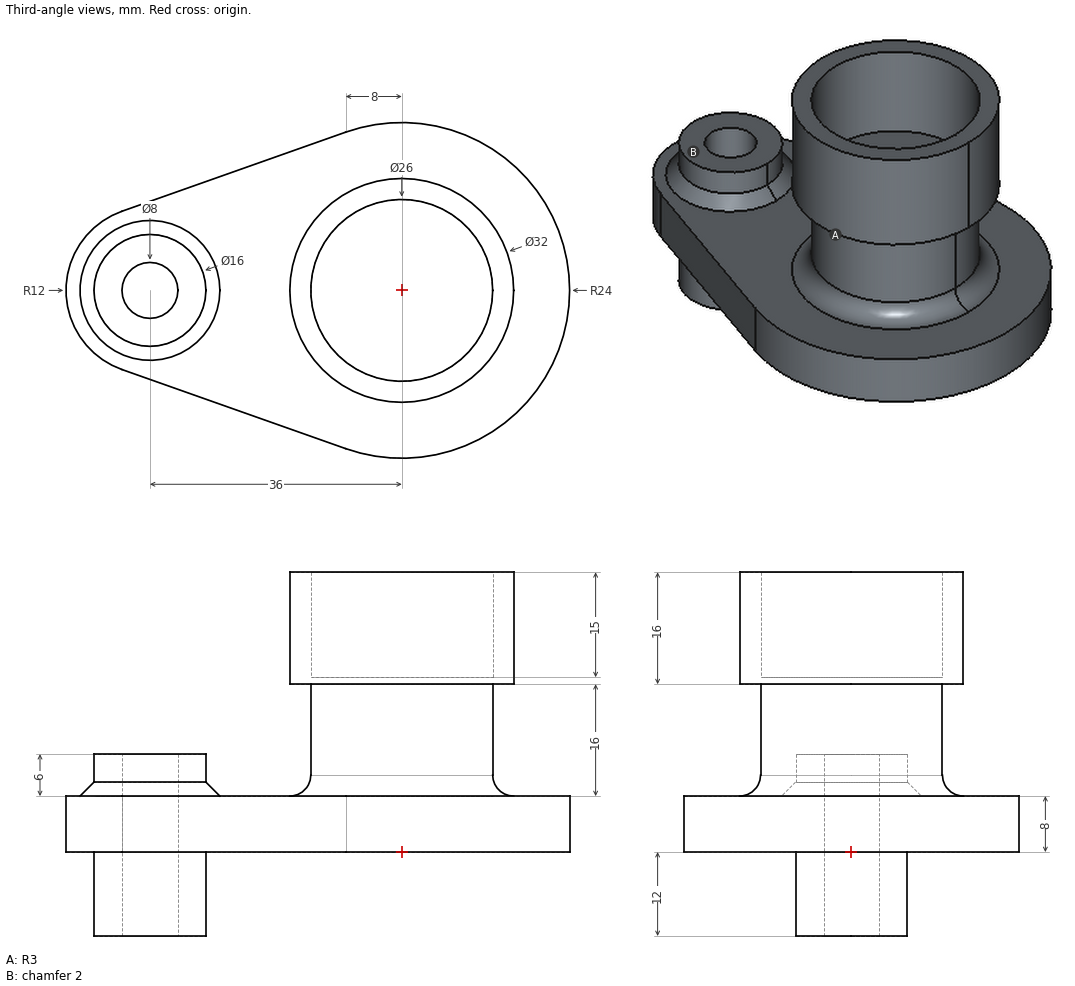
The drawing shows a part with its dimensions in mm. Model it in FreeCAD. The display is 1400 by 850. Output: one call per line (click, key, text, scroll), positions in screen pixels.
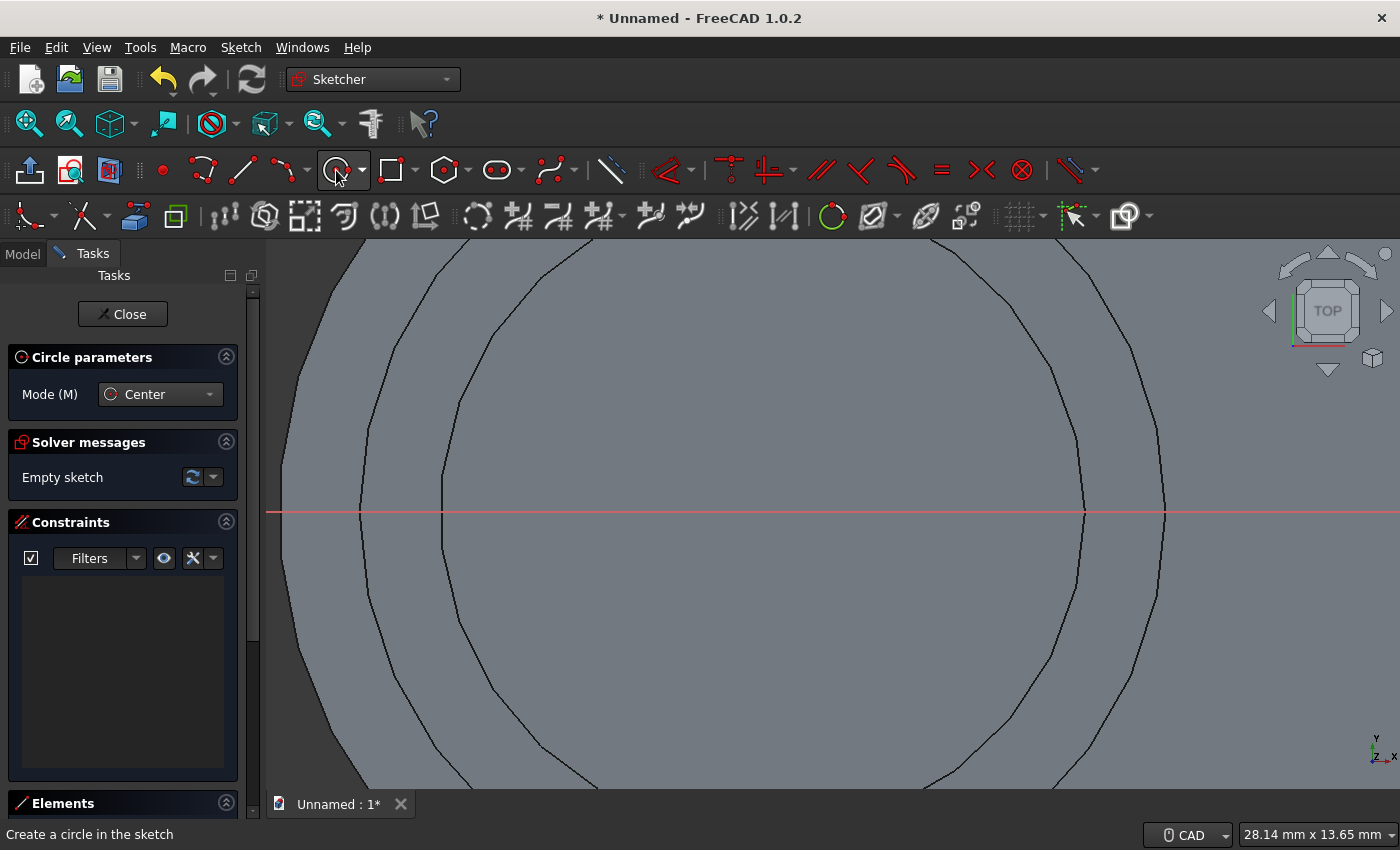
click(763, 512)
move(877, 398)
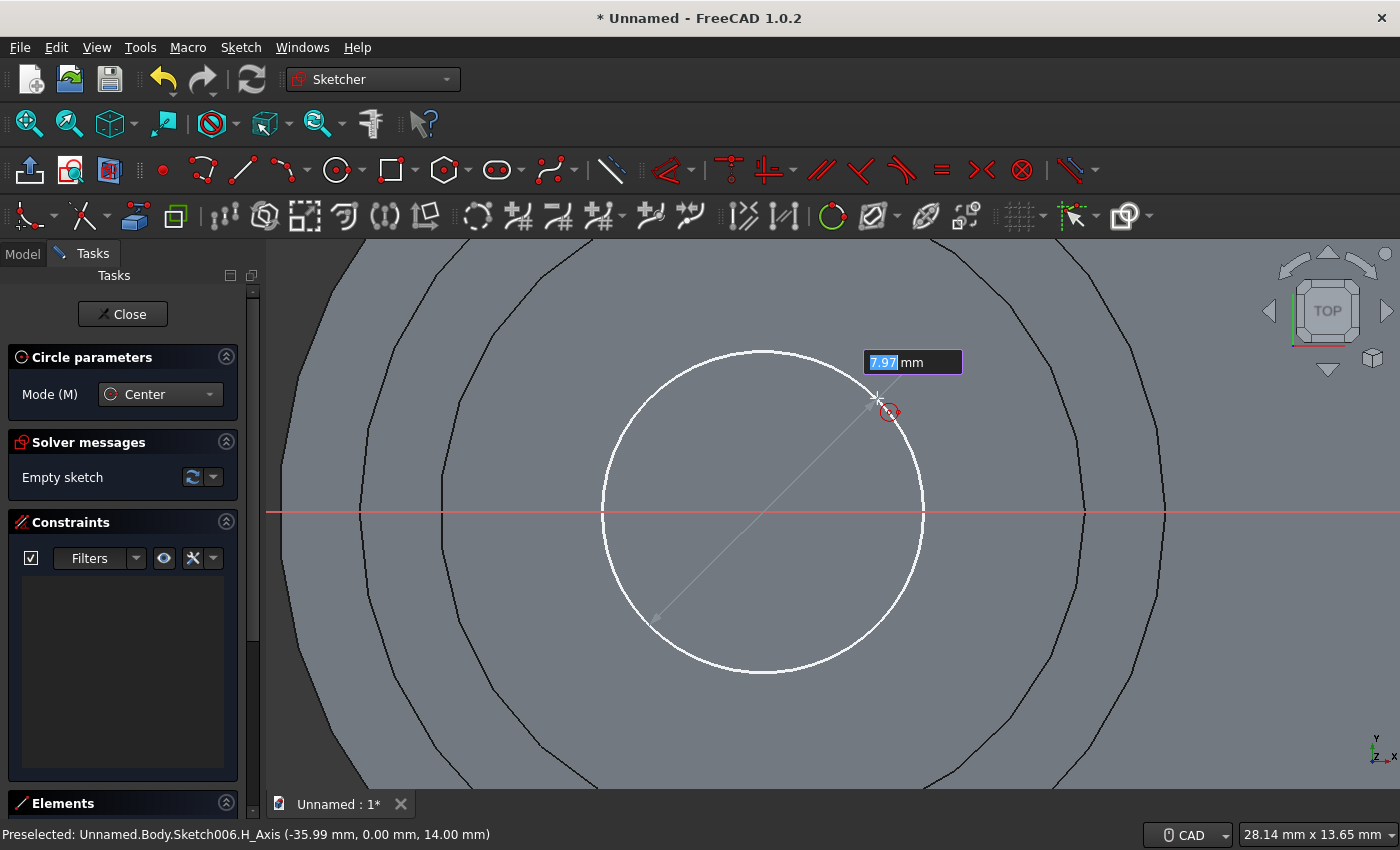
text(8)
key(Return)
key(Escape)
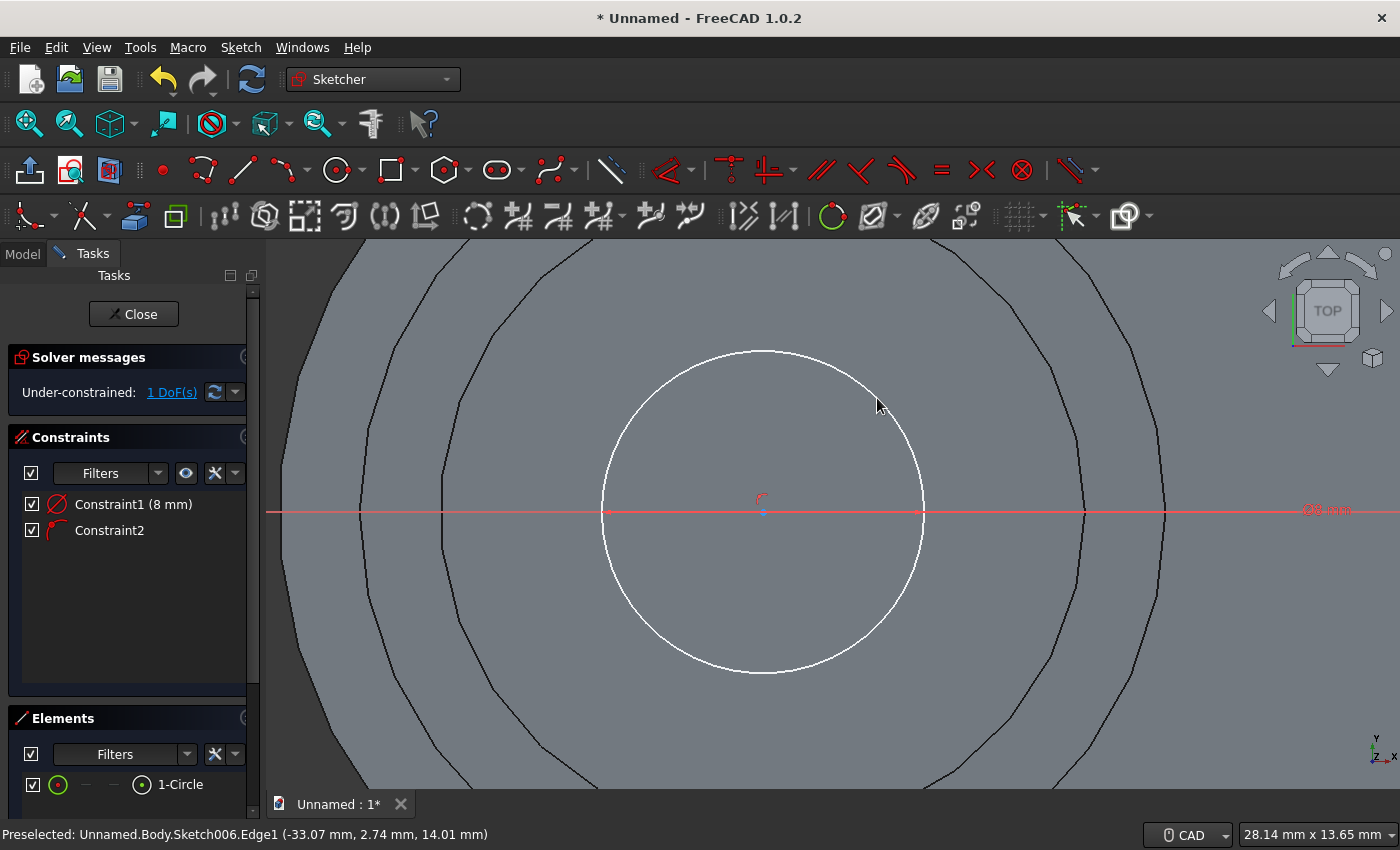
click(666, 170)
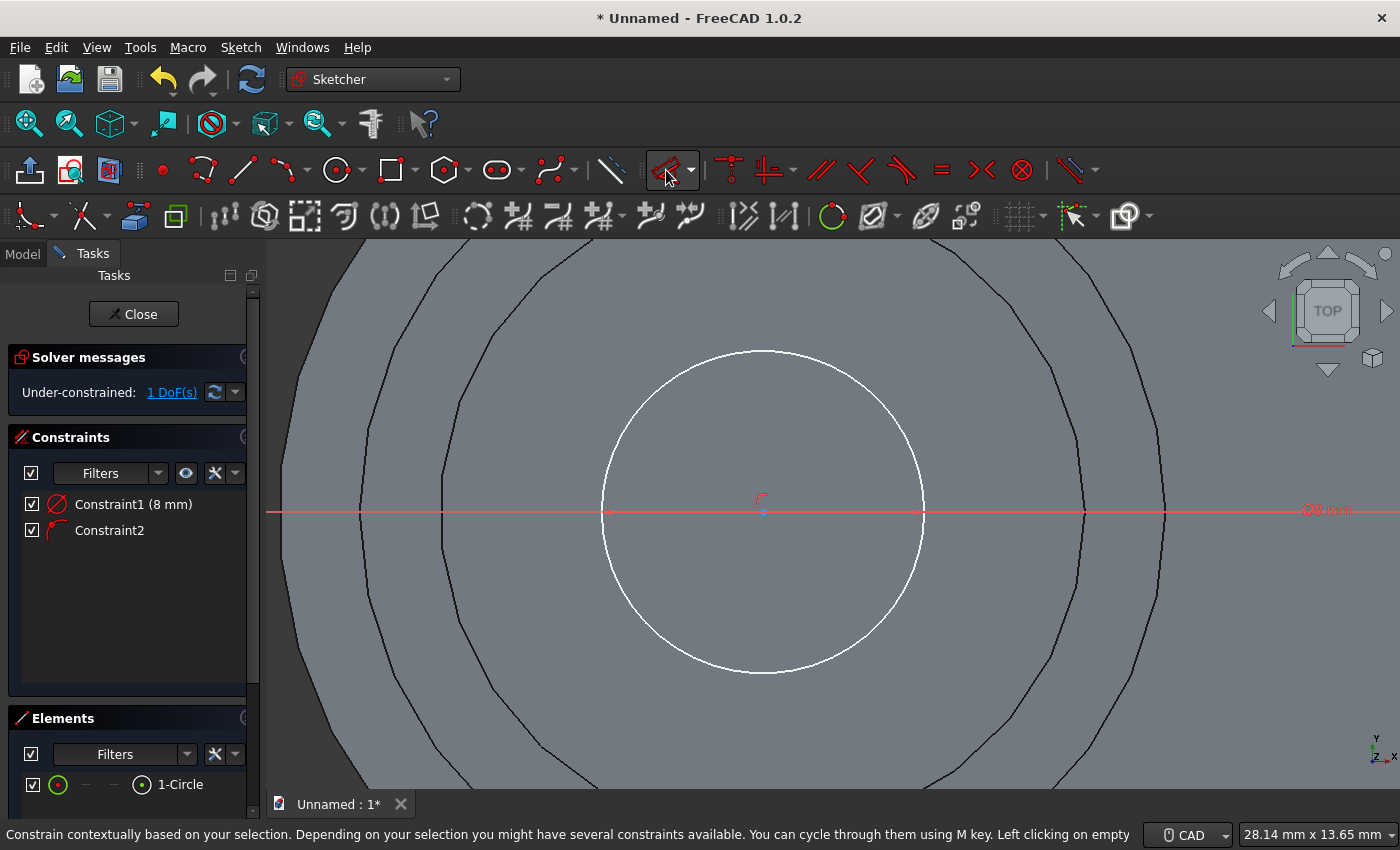
click(763, 512)
click(999, 546)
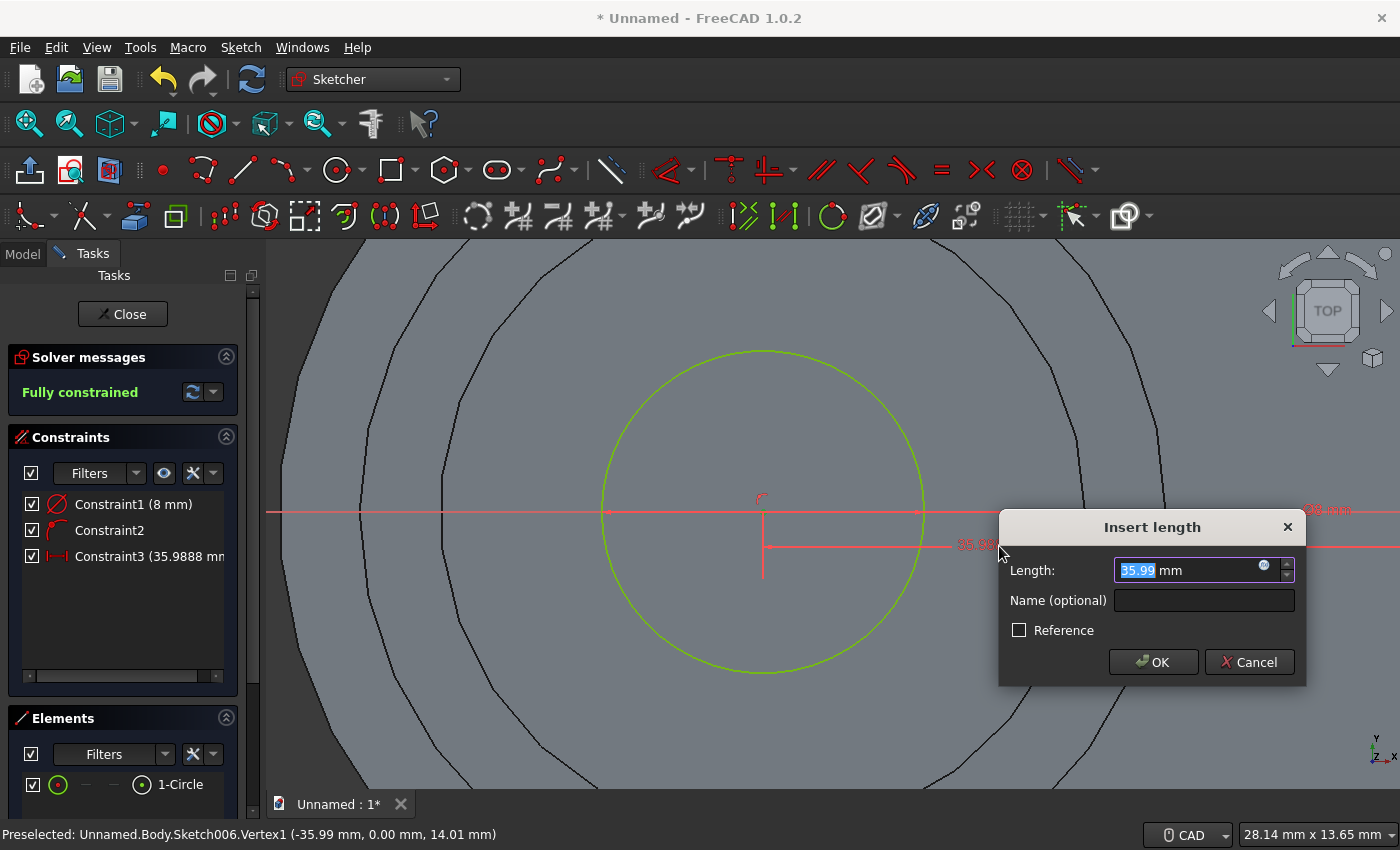
text(36)
key(Return)
key(Escape)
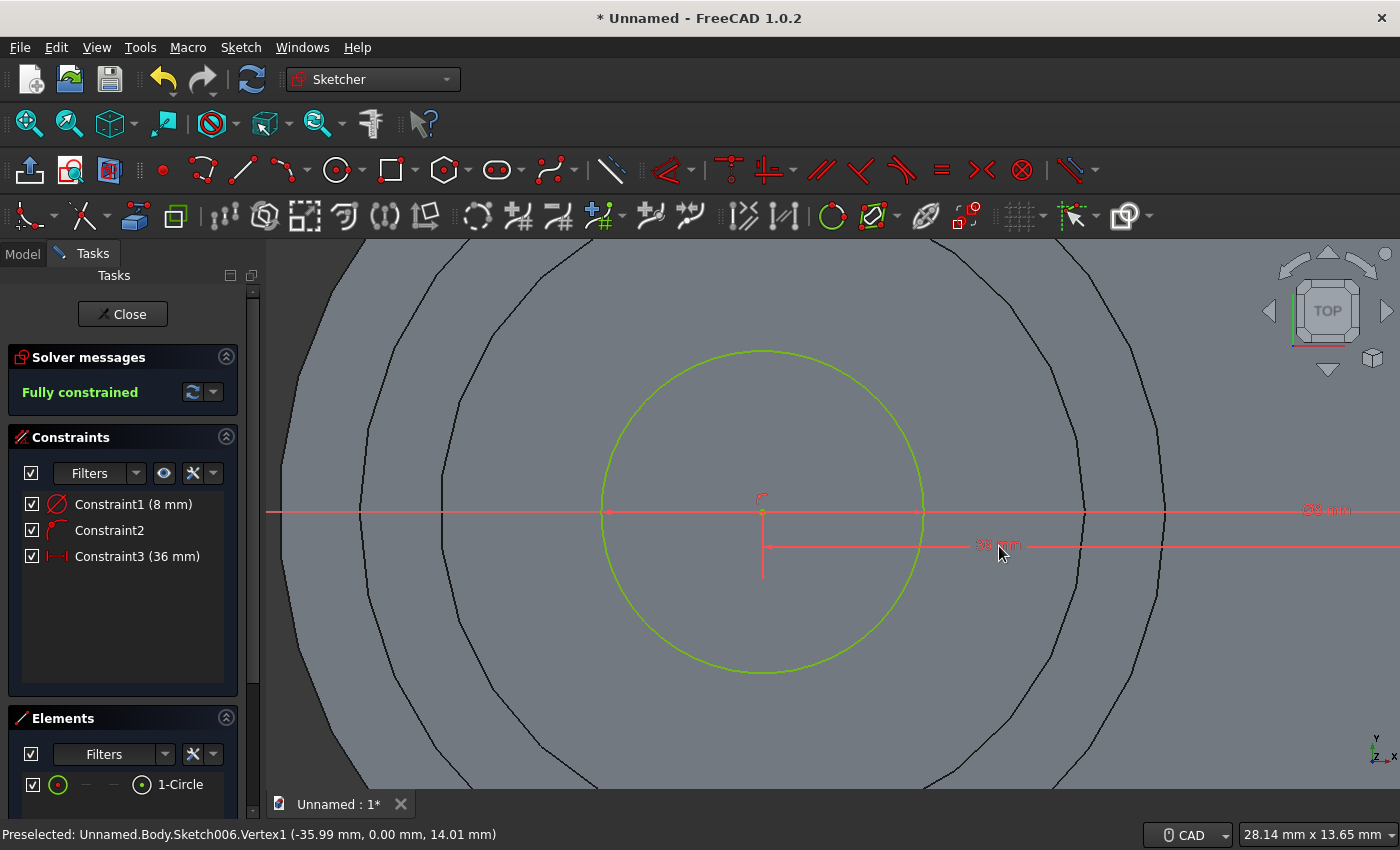
click(123, 314)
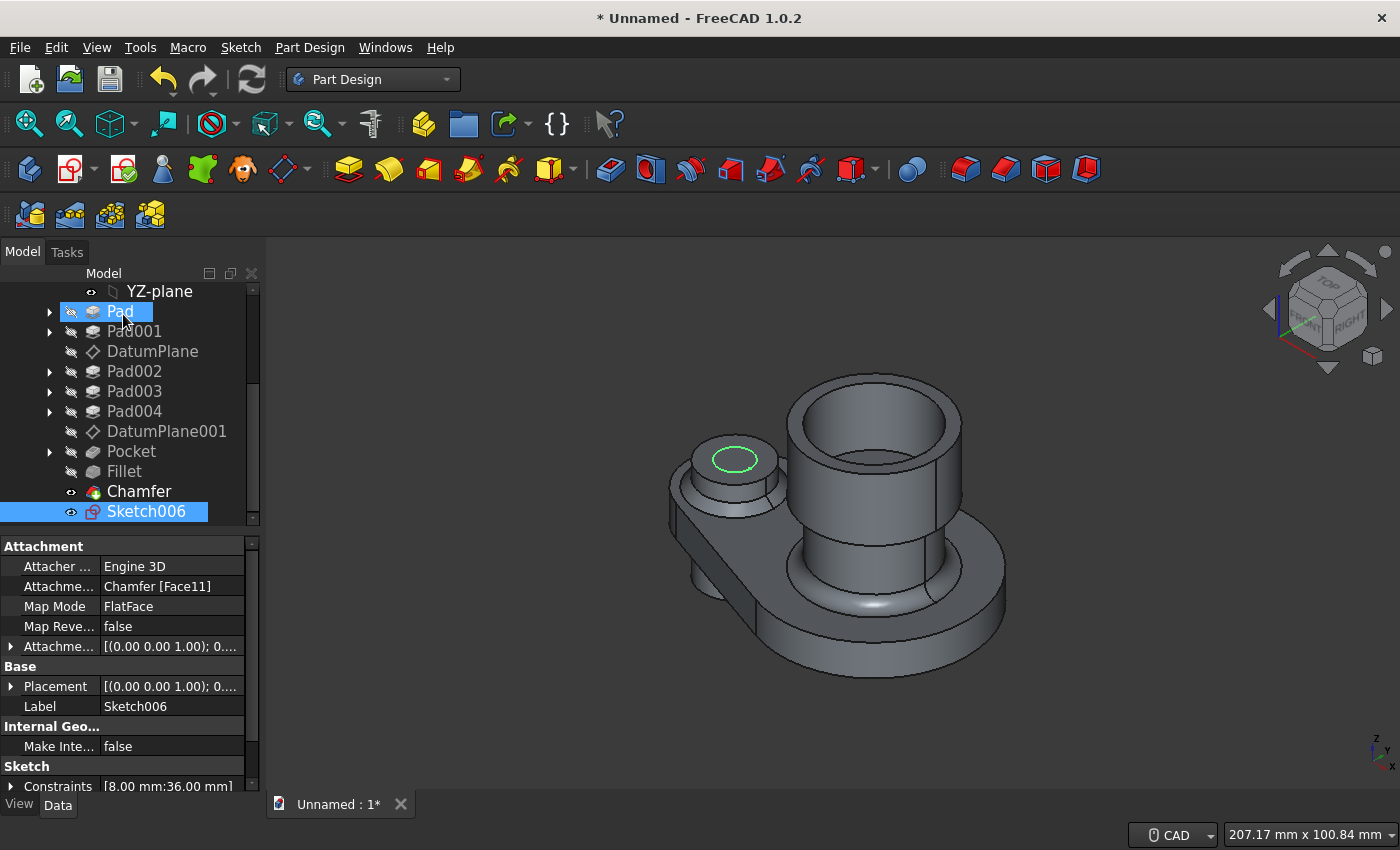
click(612, 170)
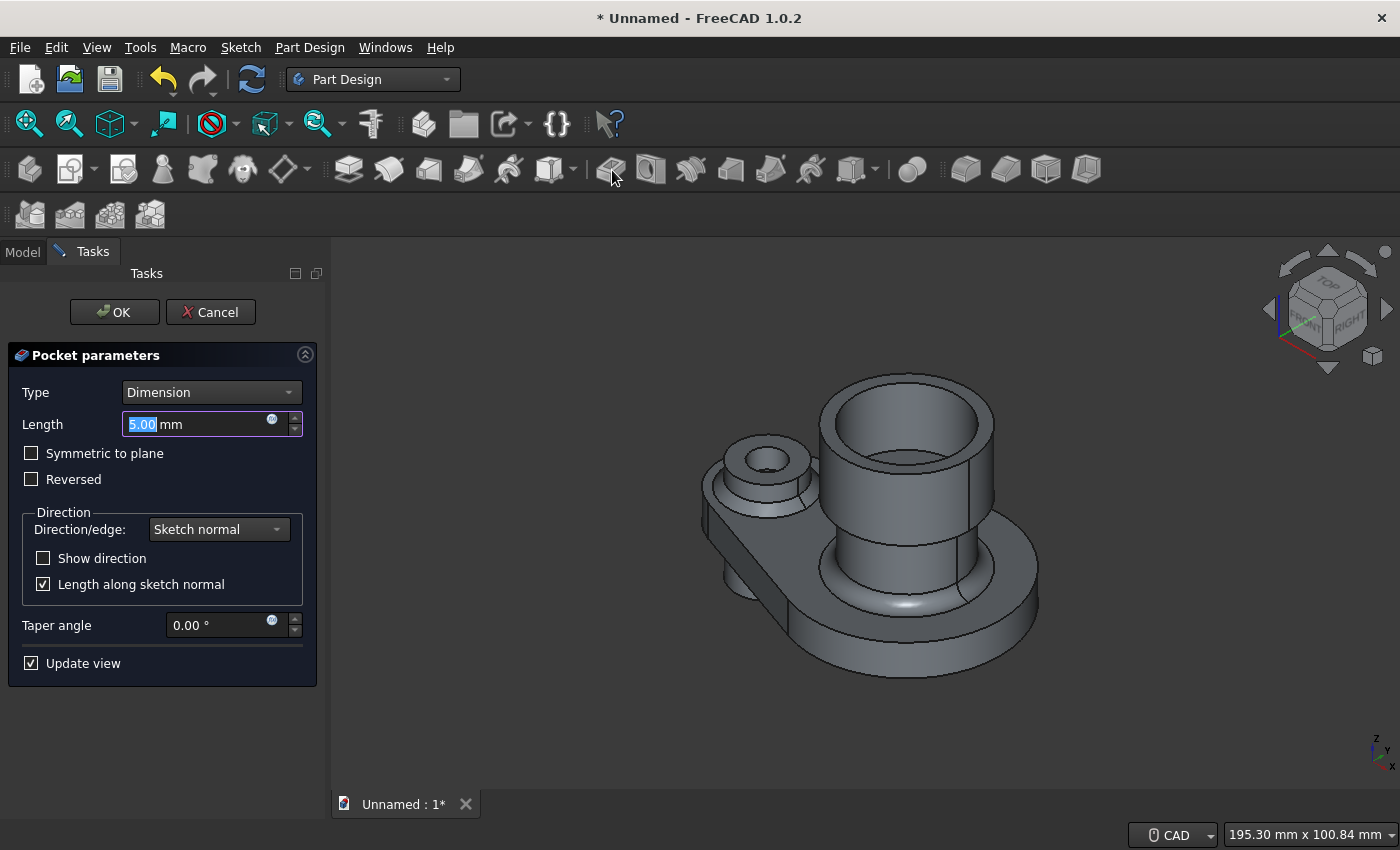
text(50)
key(Tab)